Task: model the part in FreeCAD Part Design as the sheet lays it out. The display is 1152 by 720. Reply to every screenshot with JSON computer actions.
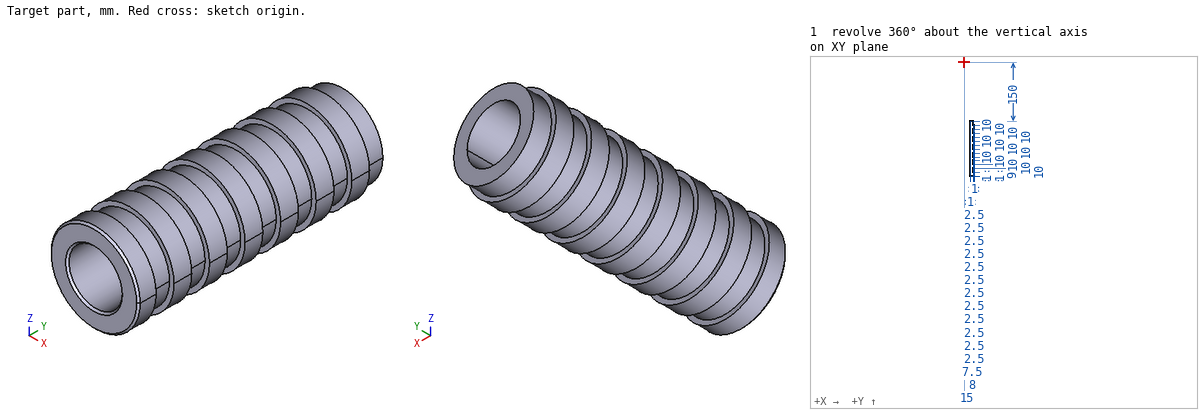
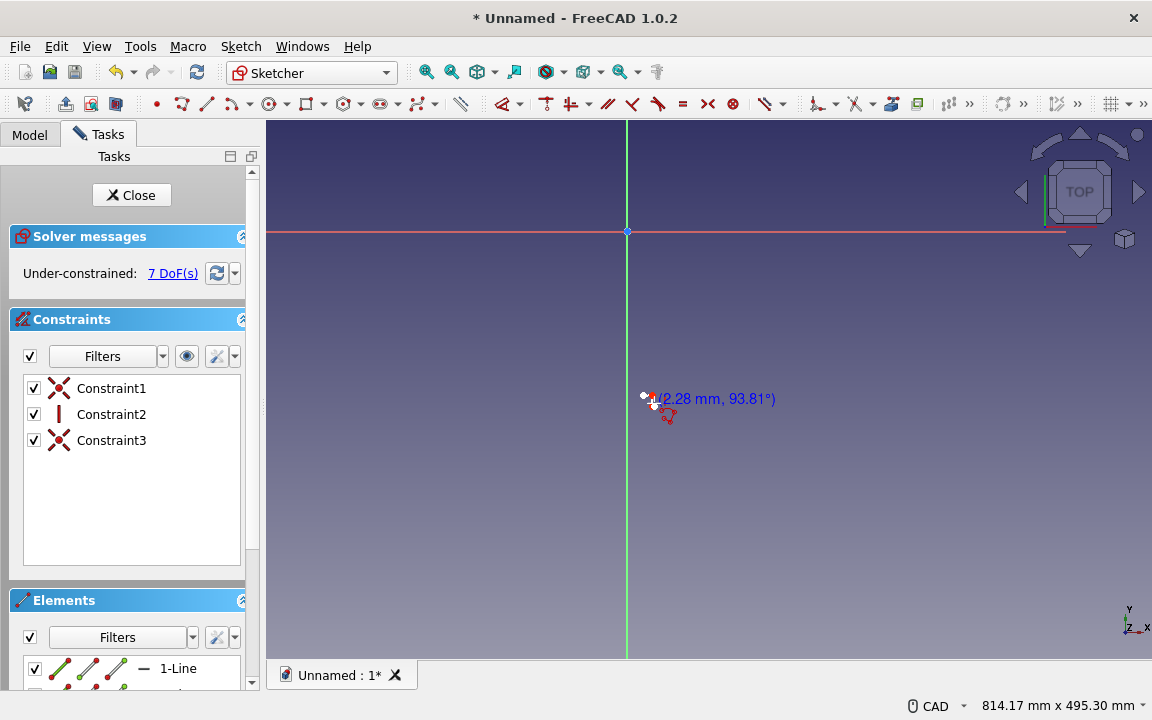
{"action": "scroll", "coordinate": [655, 417], "scroll_direction": "up", "scroll_amount": 2}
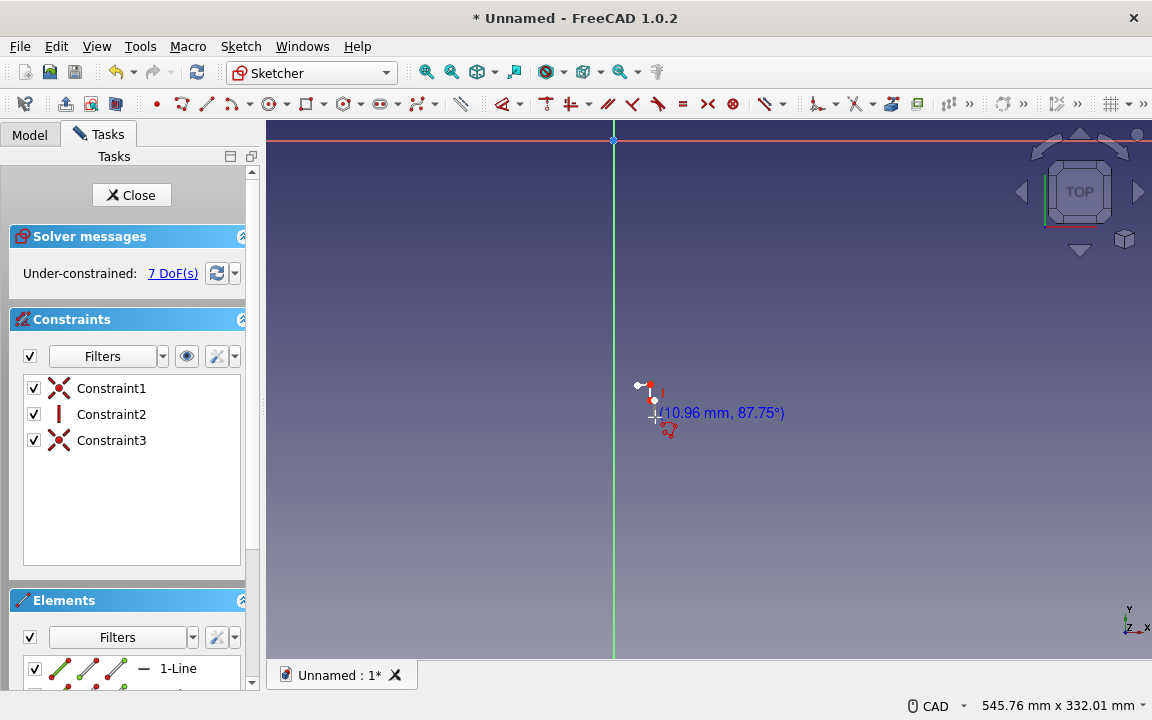
{"action": "left_click", "coordinate": [654, 416]}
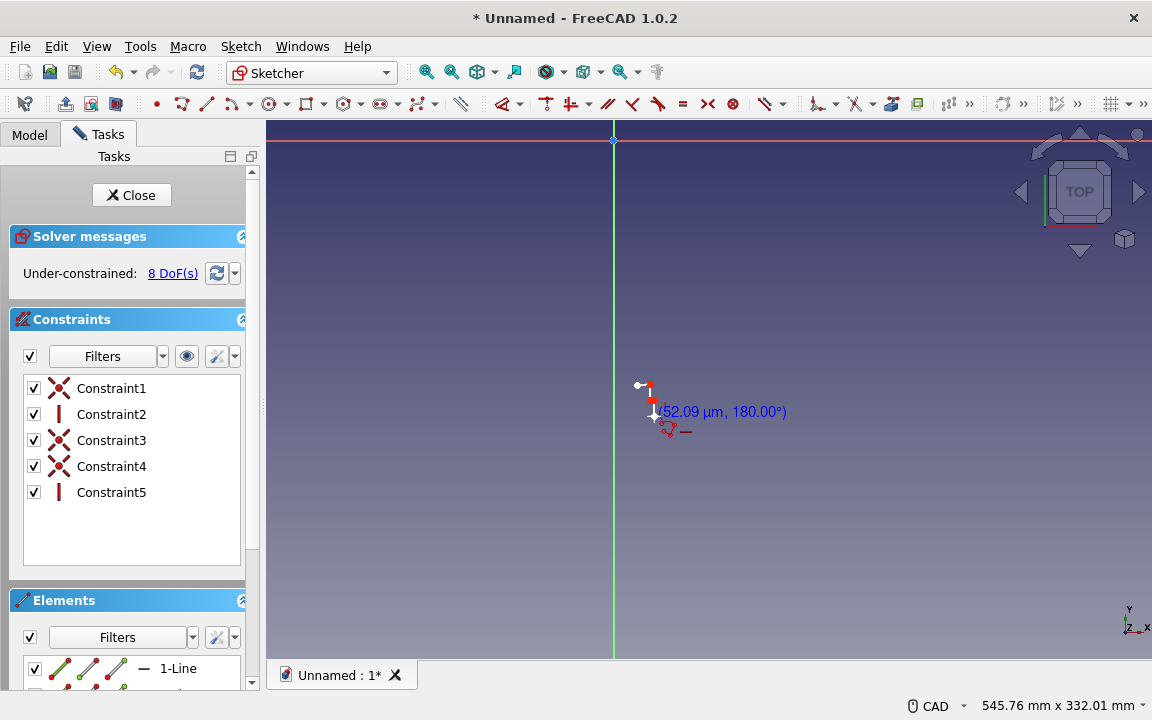
{"action": "scroll", "coordinate": [650, 416], "scroll_direction": "up", "scroll_amount": 7}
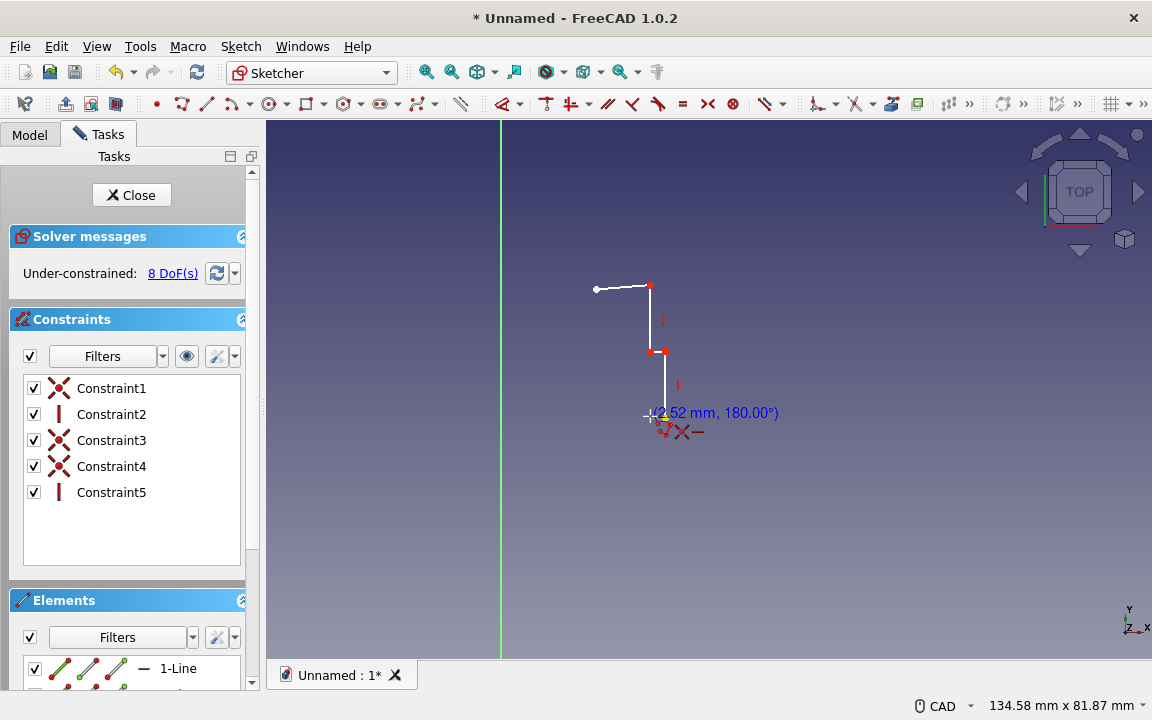
{"action": "left_click", "coordinate": [649, 414]}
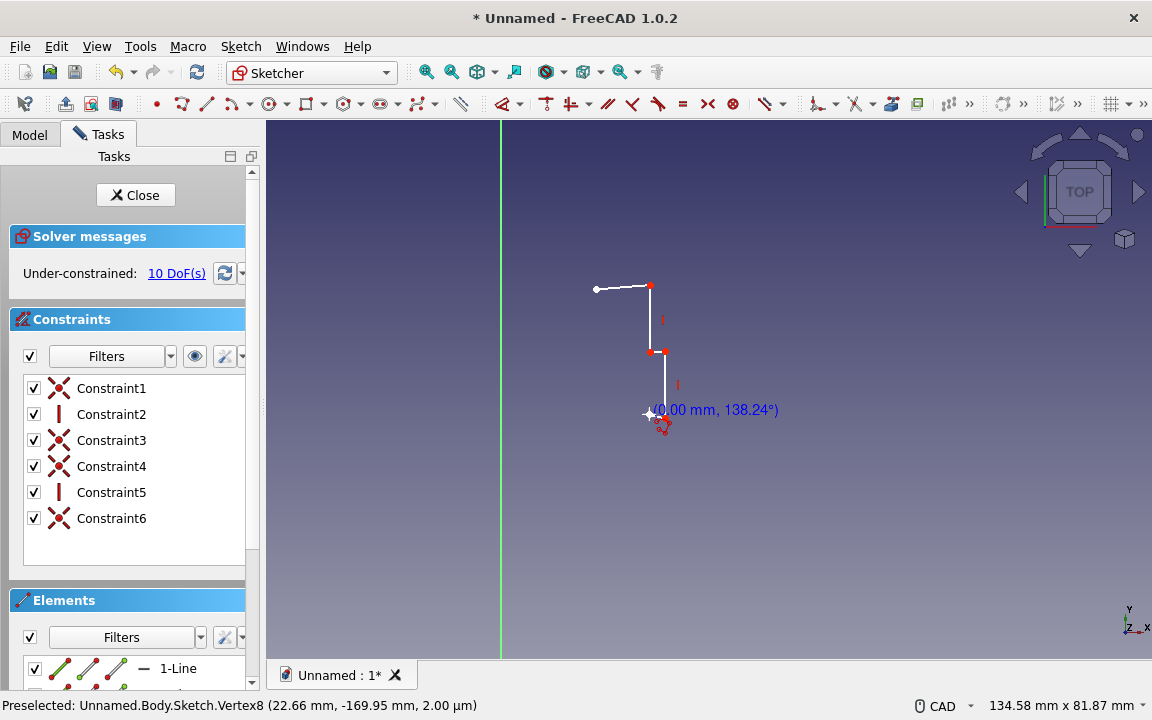
{"action": "scroll", "coordinate": [652, 417], "scroll_direction": "down", "scroll_amount": 9}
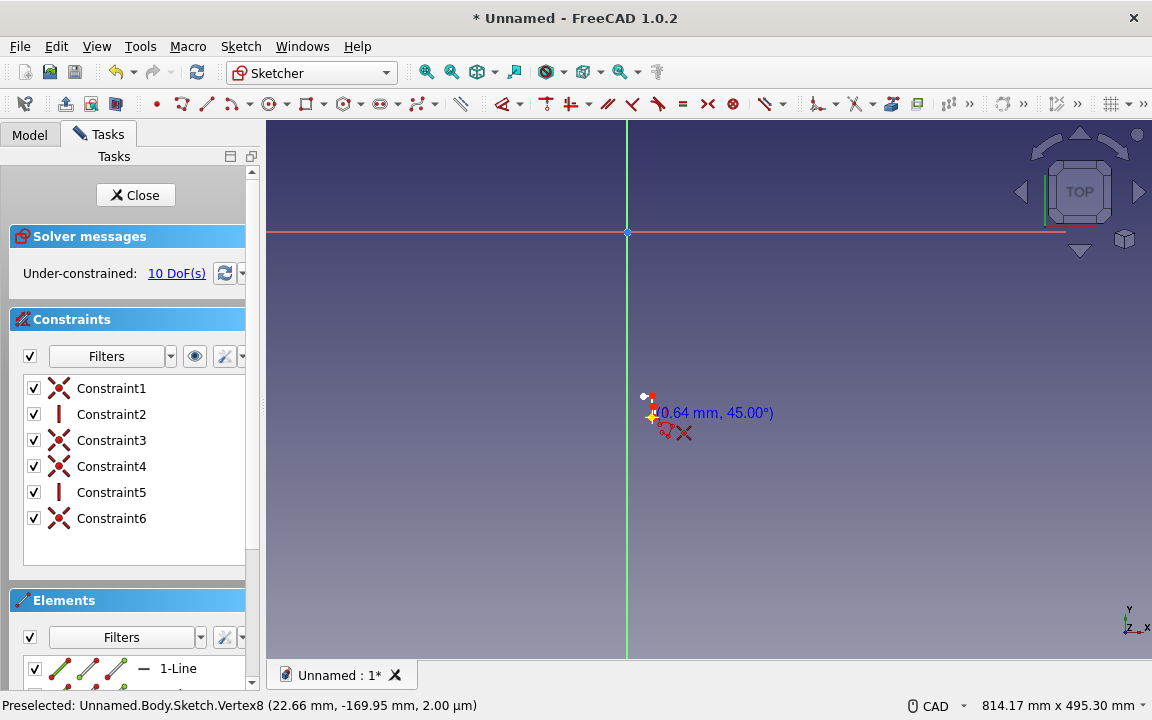
{"action": "scroll", "coordinate": [652, 428], "scroll_direction": "up", "scroll_amount": 2}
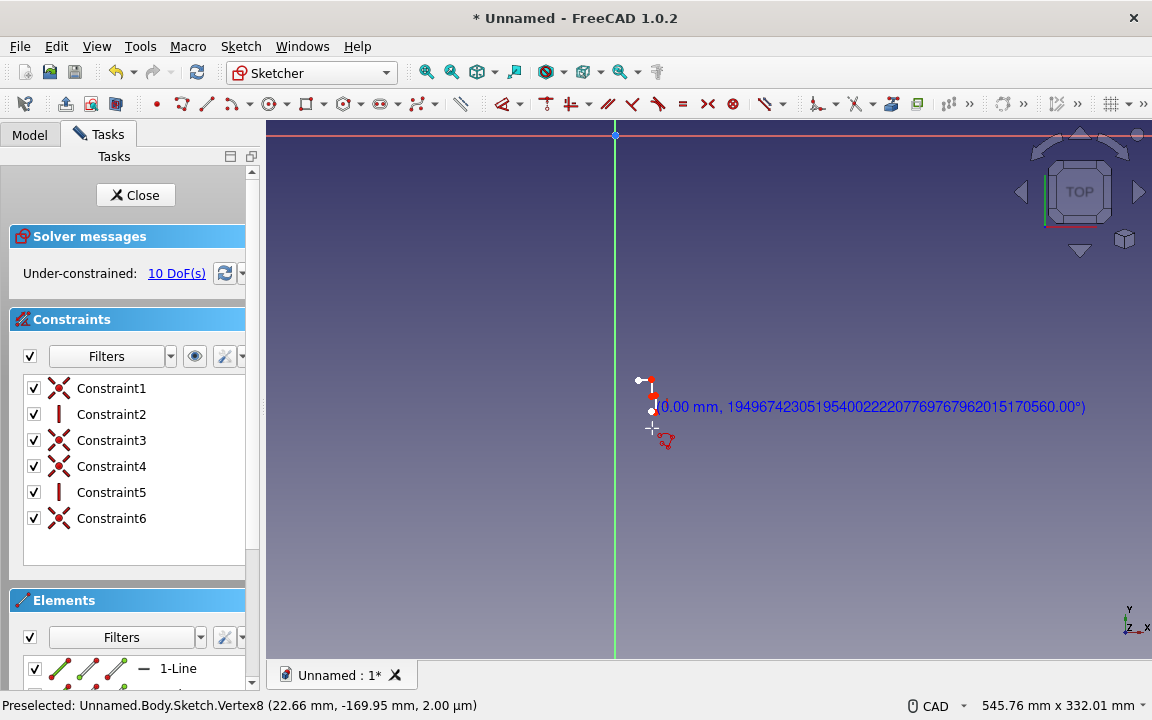
{"action": "left_click", "coordinate": [652, 428]}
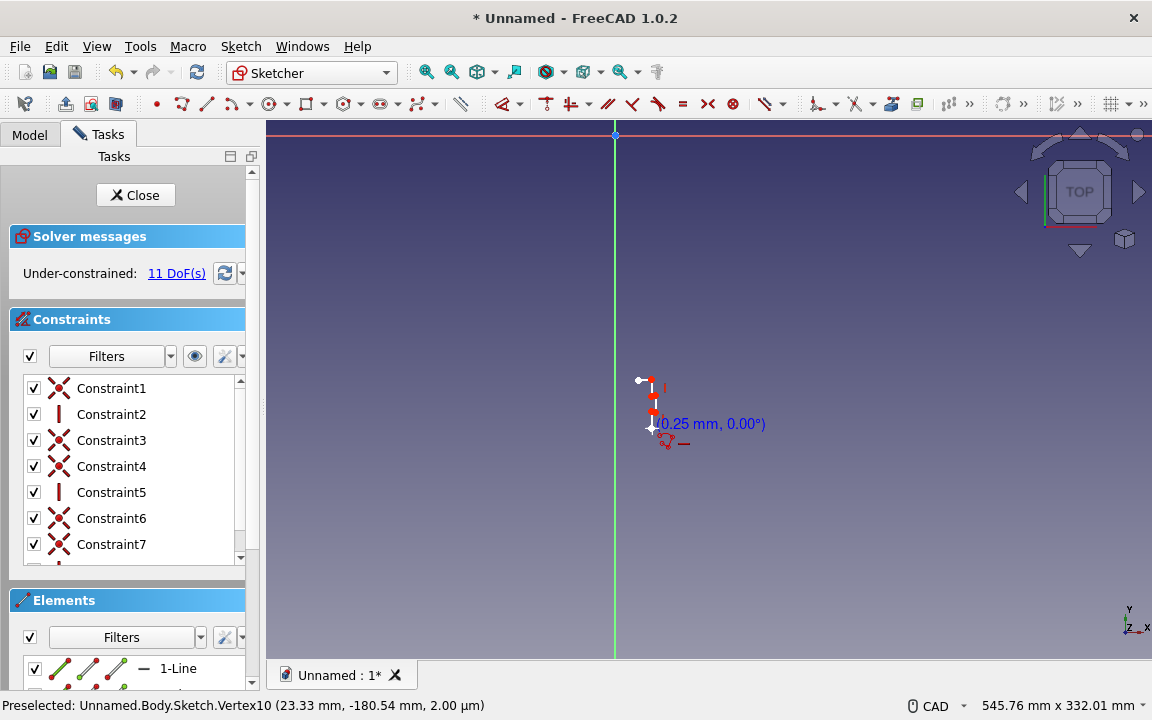
{"action": "scroll", "coordinate": [656, 428], "scroll_direction": "up", "scroll_amount": 7}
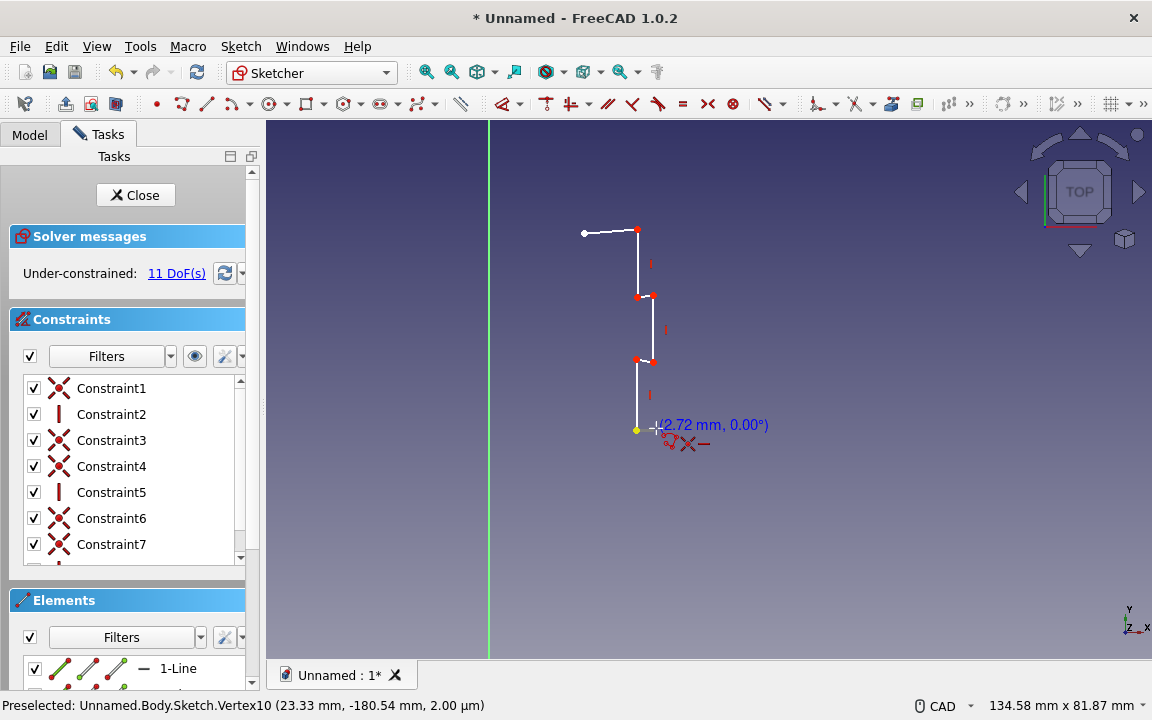
{"action": "left_click", "coordinate": [653, 426]}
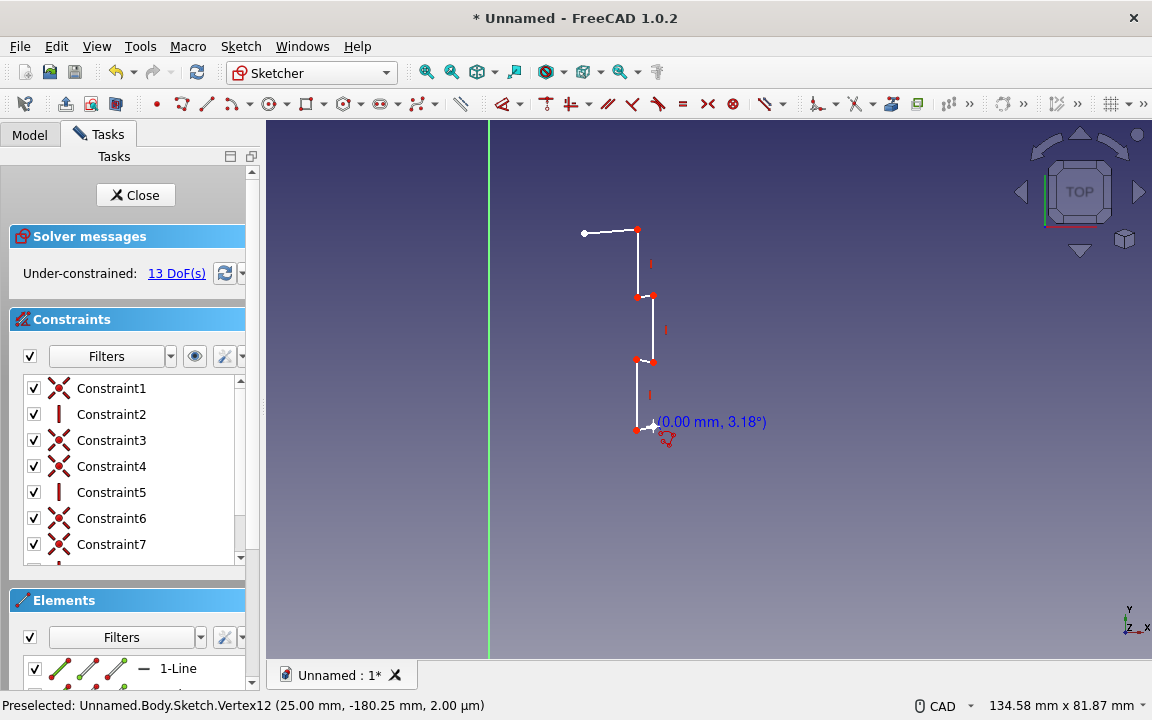
{"action": "scroll", "coordinate": [654, 428], "scroll_direction": "down", "scroll_amount": 9}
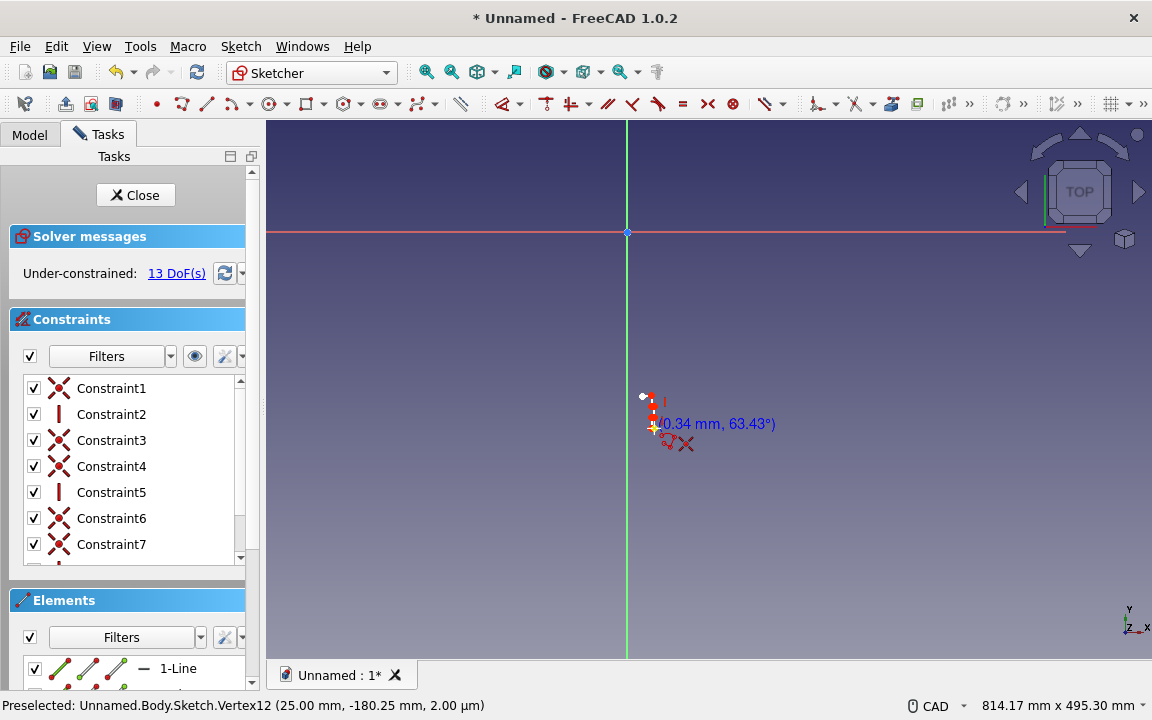
{"action": "scroll", "coordinate": [654, 439], "scroll_direction": "up", "scroll_amount": 2}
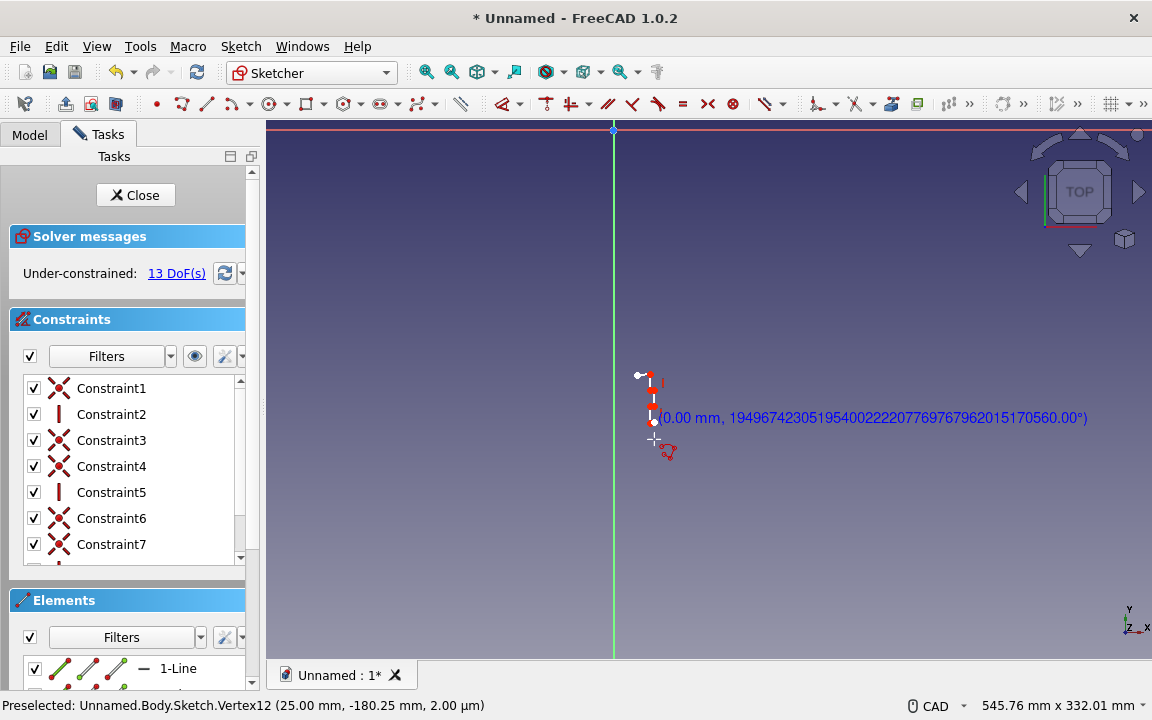
{"action": "left_click", "coordinate": [654, 439]}